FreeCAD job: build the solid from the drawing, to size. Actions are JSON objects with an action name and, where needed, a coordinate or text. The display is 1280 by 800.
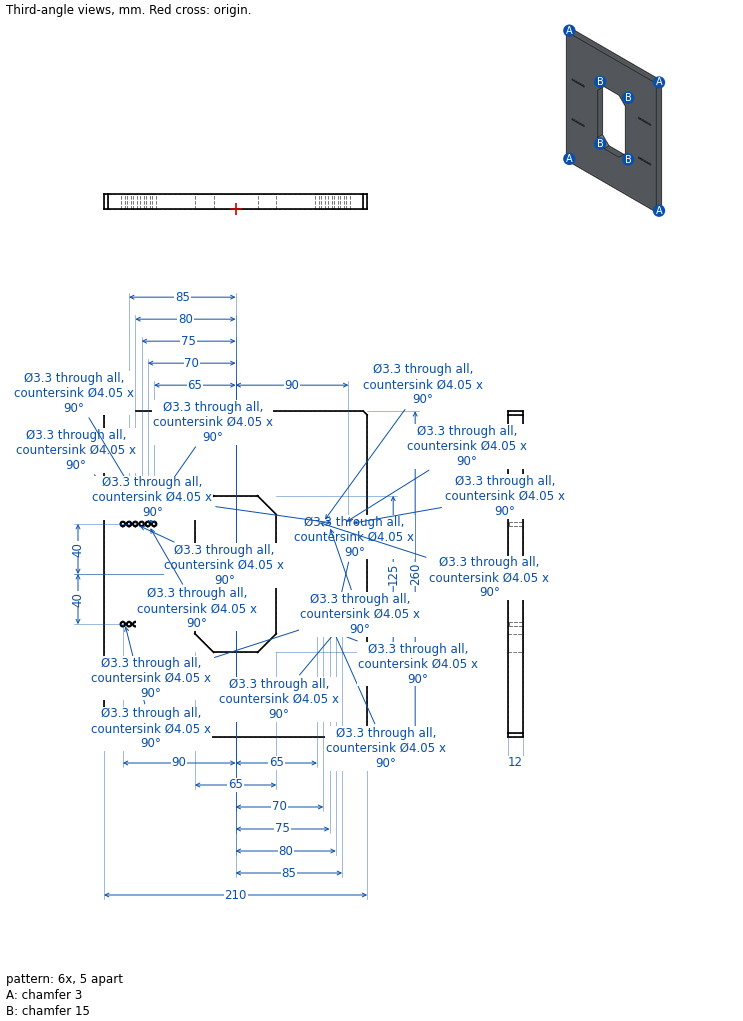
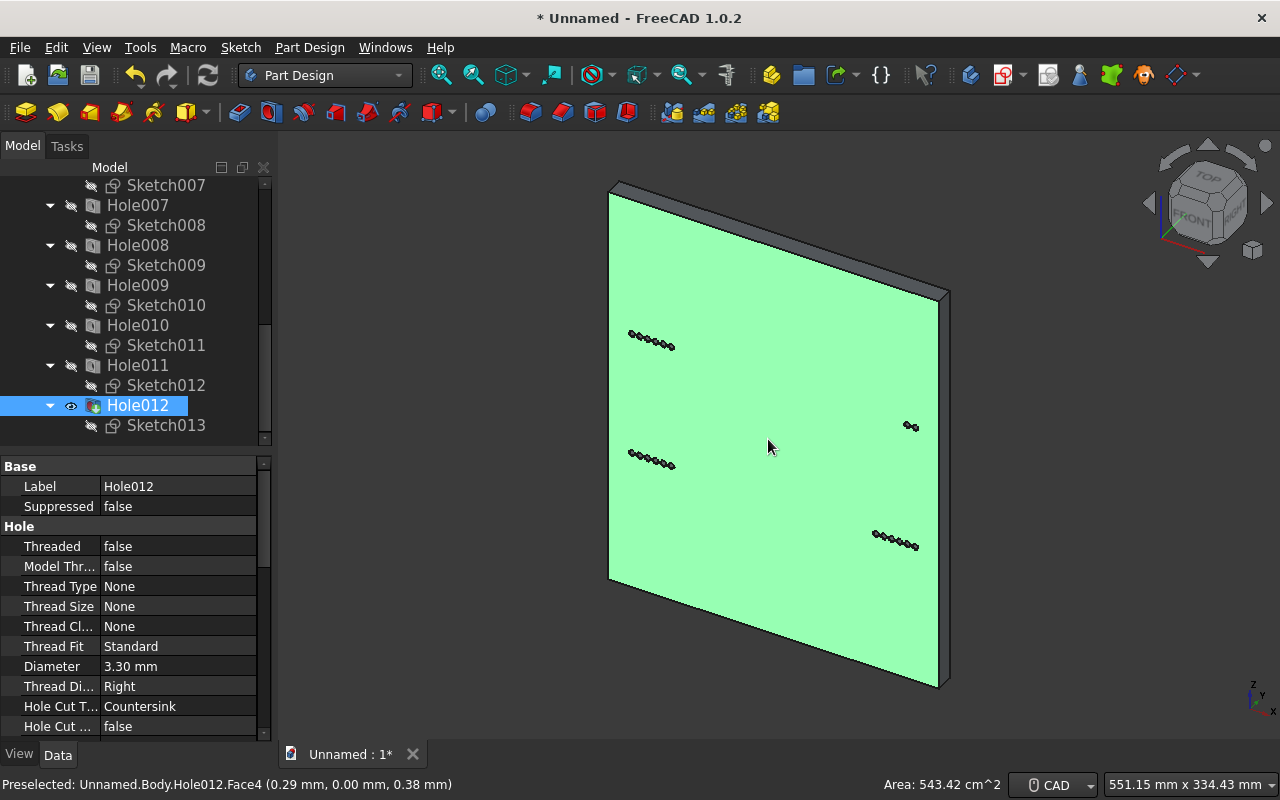
{"action": "left_click", "coordinate": [1004, 76]}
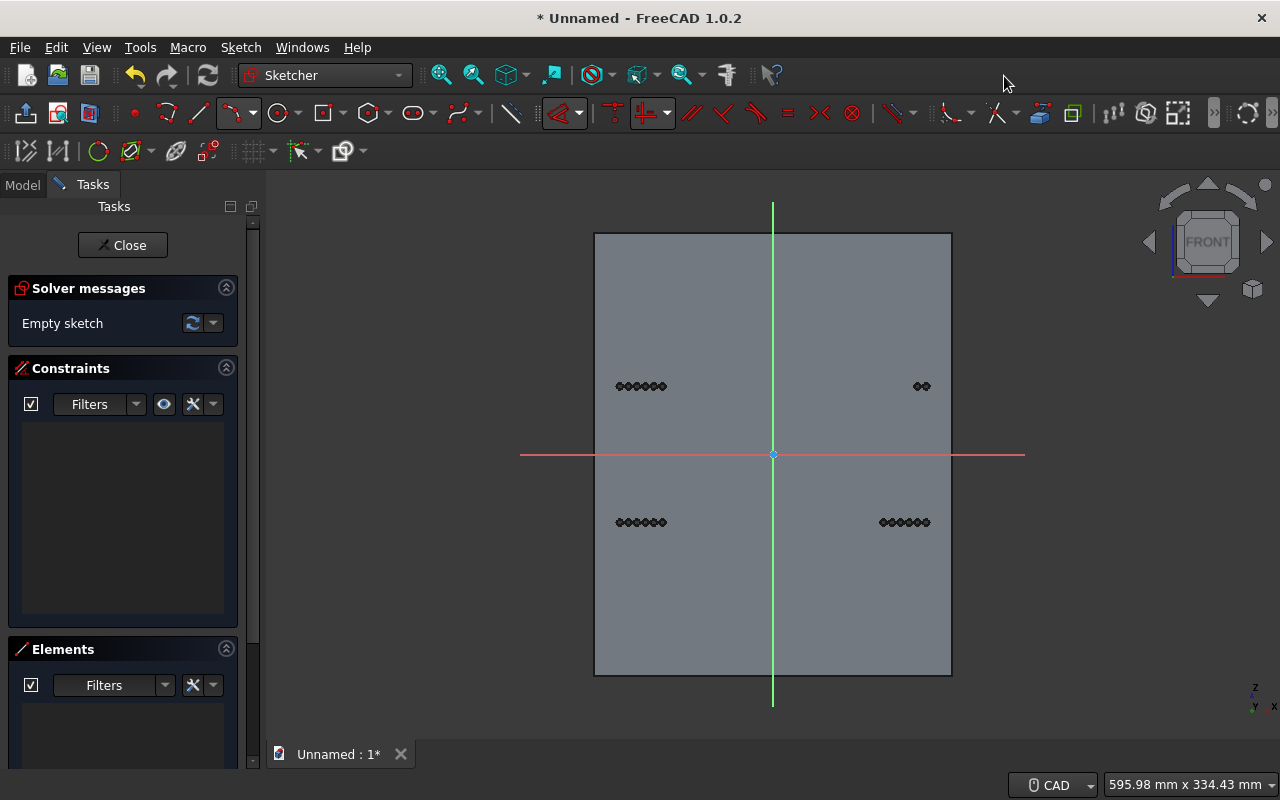
{"action": "scroll", "coordinate": [920, 383], "scroll_direction": "up", "scroll_amount": 15}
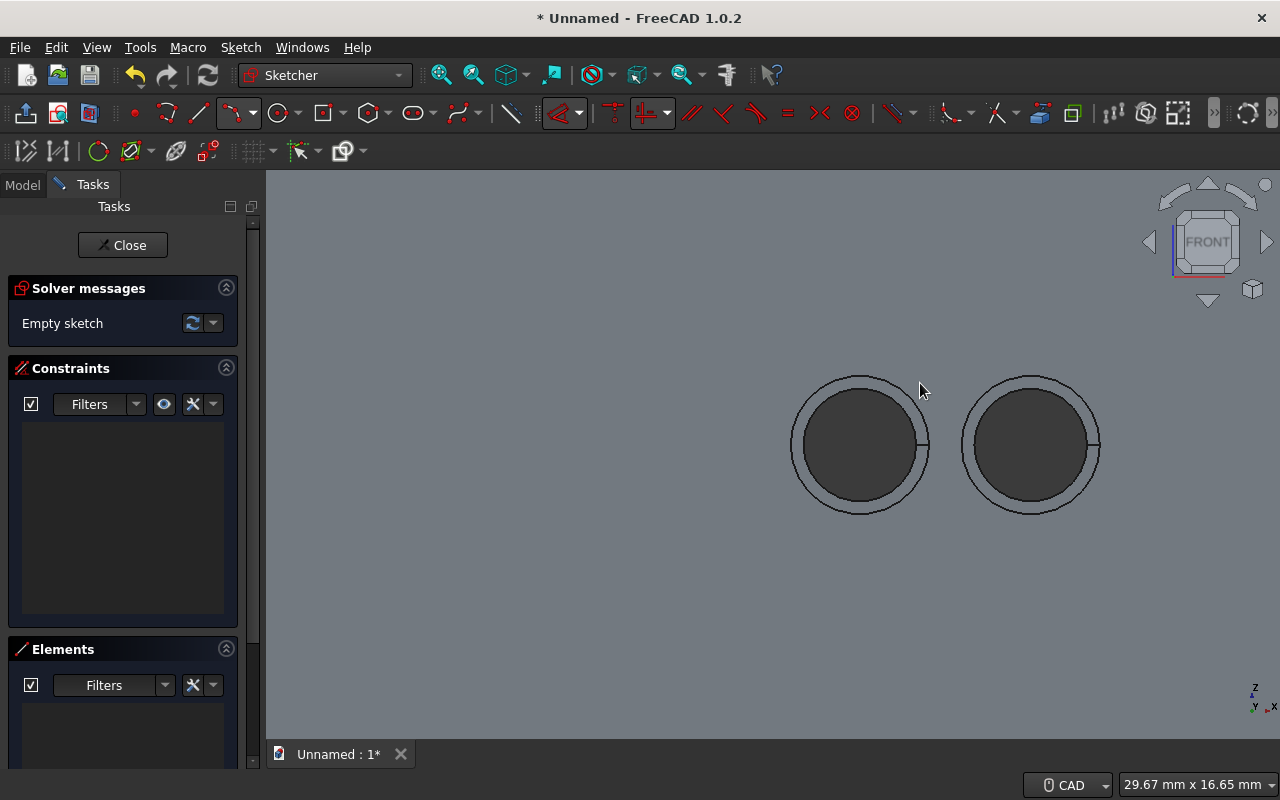
{"action": "scroll", "coordinate": [682, 441], "scroll_direction": "up", "scroll_amount": 6}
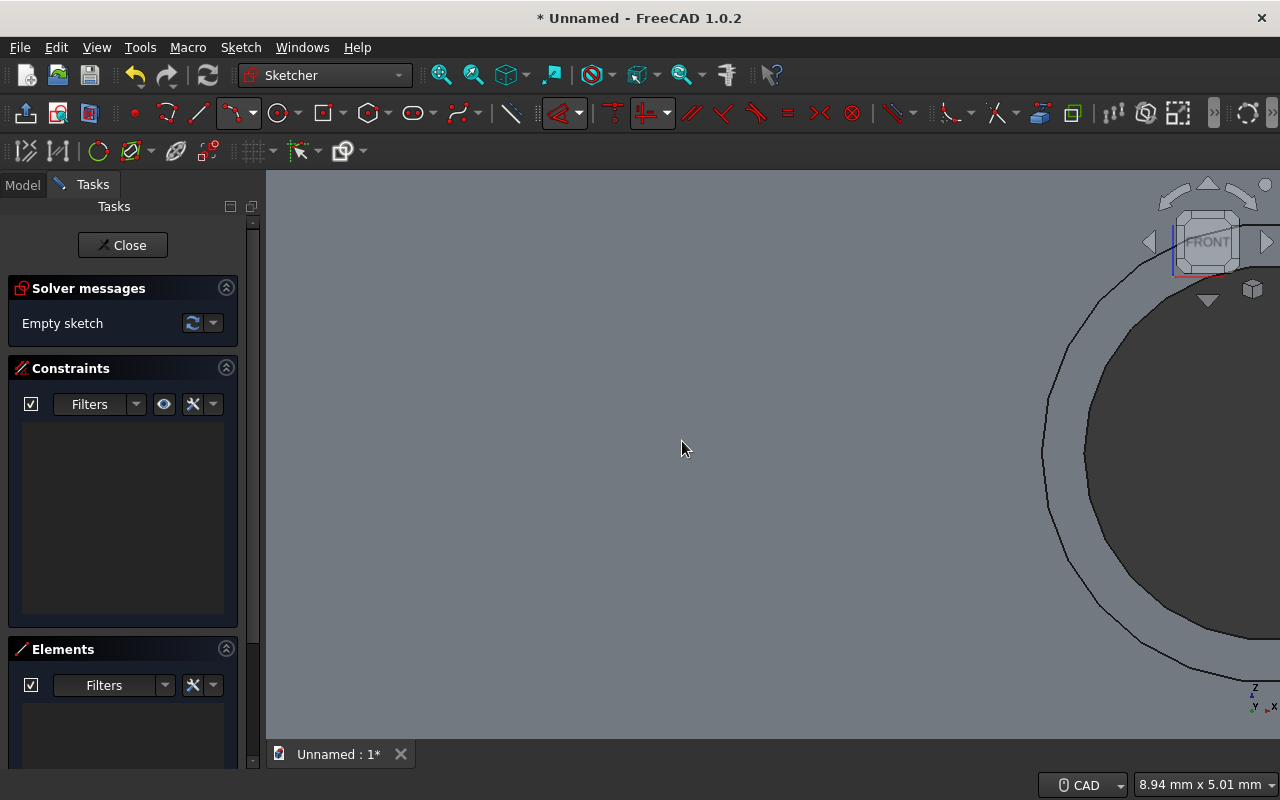
{"action": "left_click", "coordinate": [278, 114]}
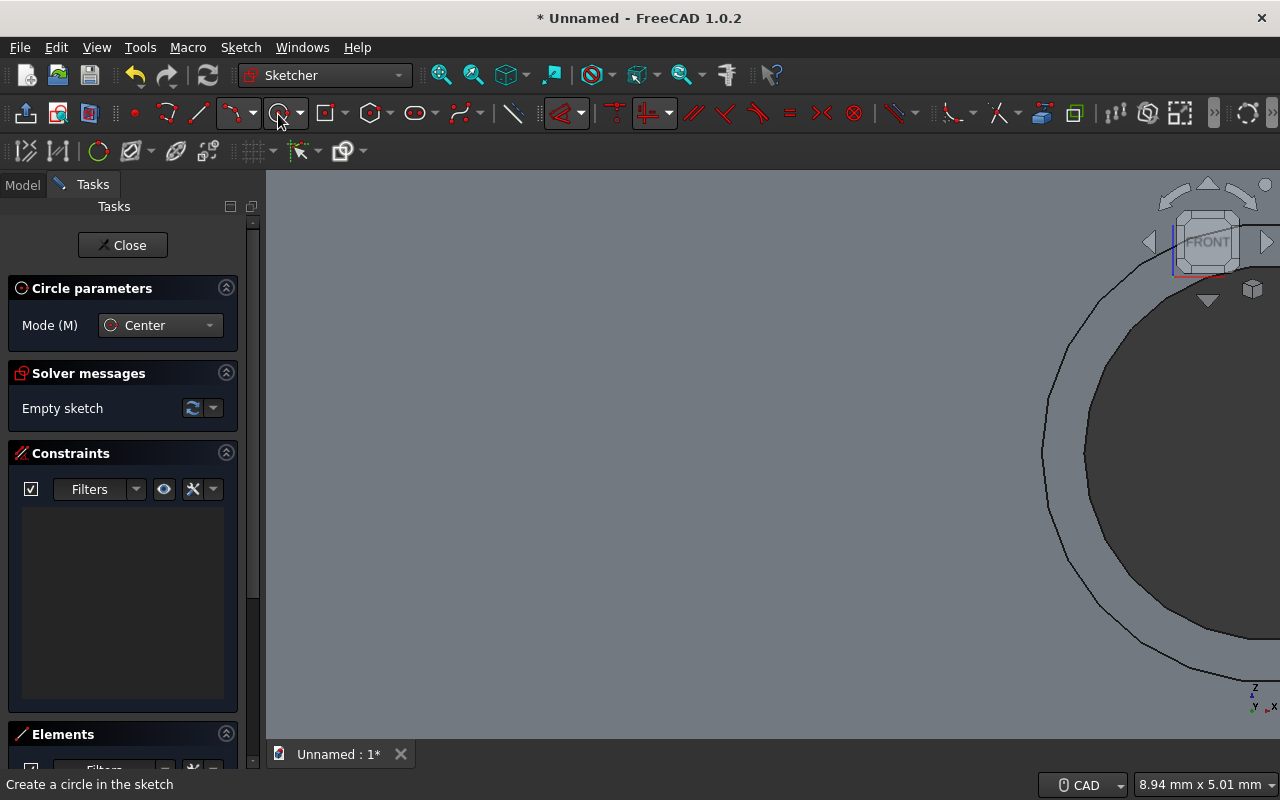
{"action": "left_click", "coordinate": [704, 453]}
{"action": "mouse_move", "coordinate": [837, 321]}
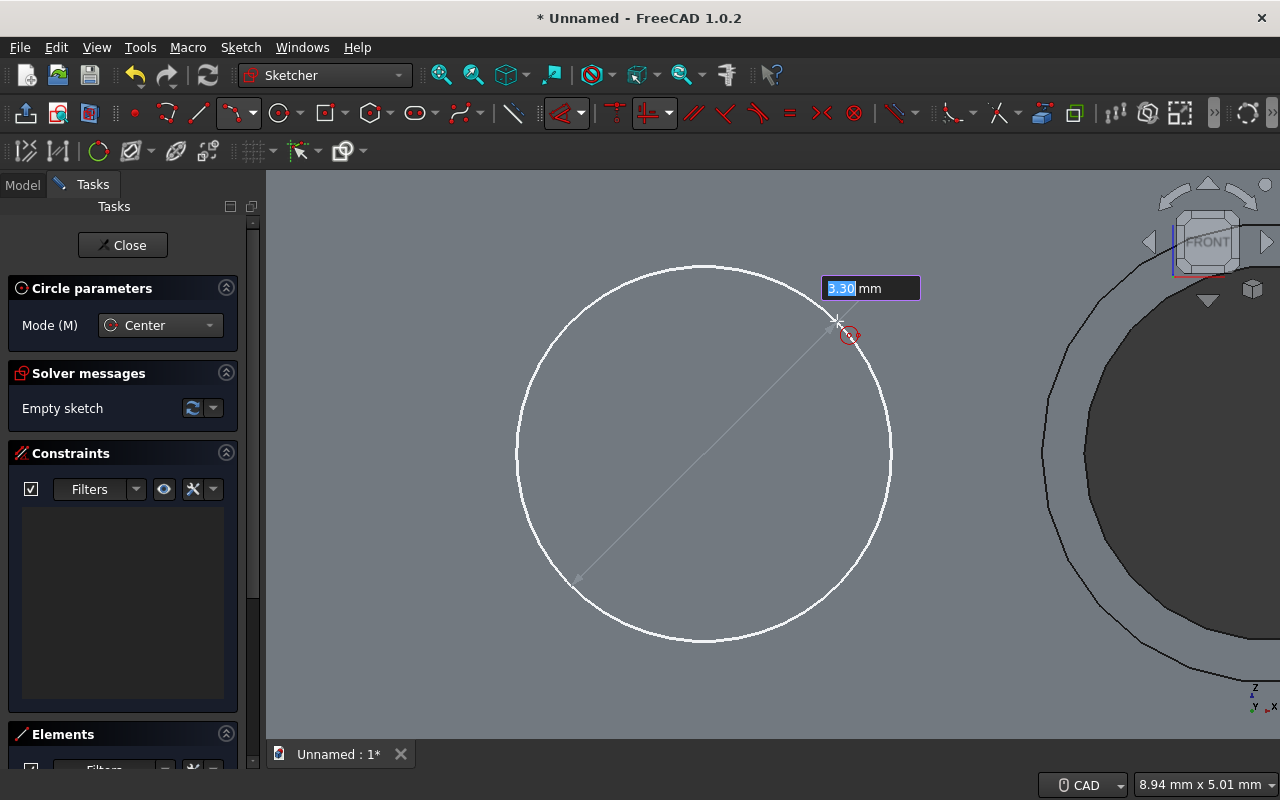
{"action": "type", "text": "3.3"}
{"action": "key", "text": "Return"}
{"action": "key", "text": "Escape"}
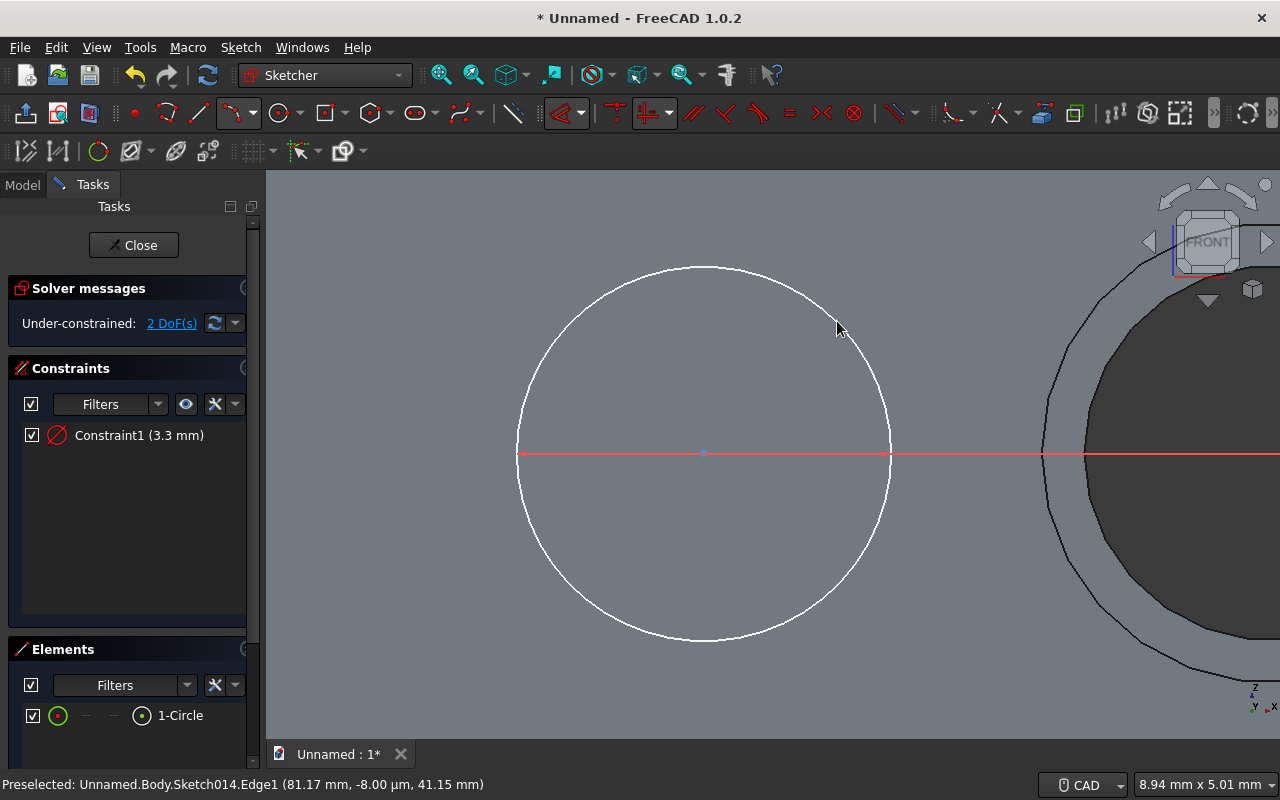
{"action": "left_click", "coordinate": [704, 454]}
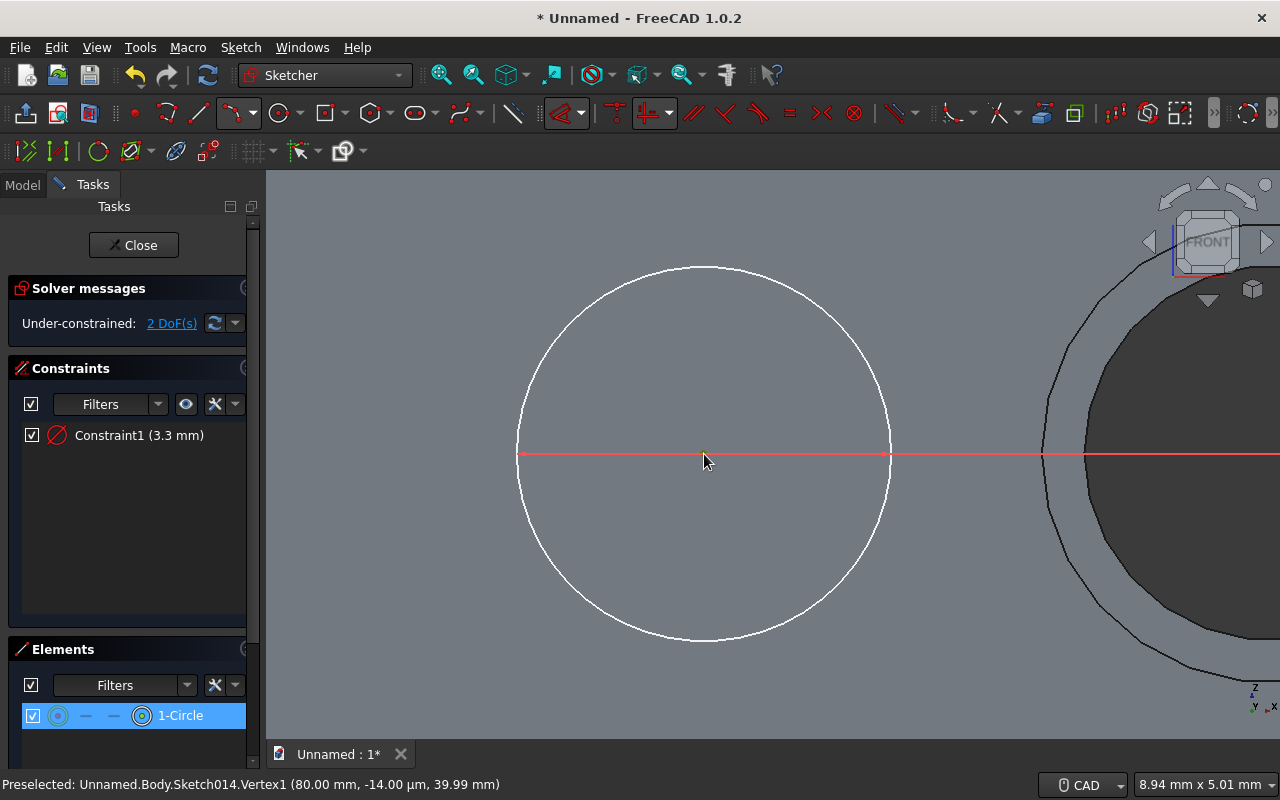
{"action": "key", "text": "l"}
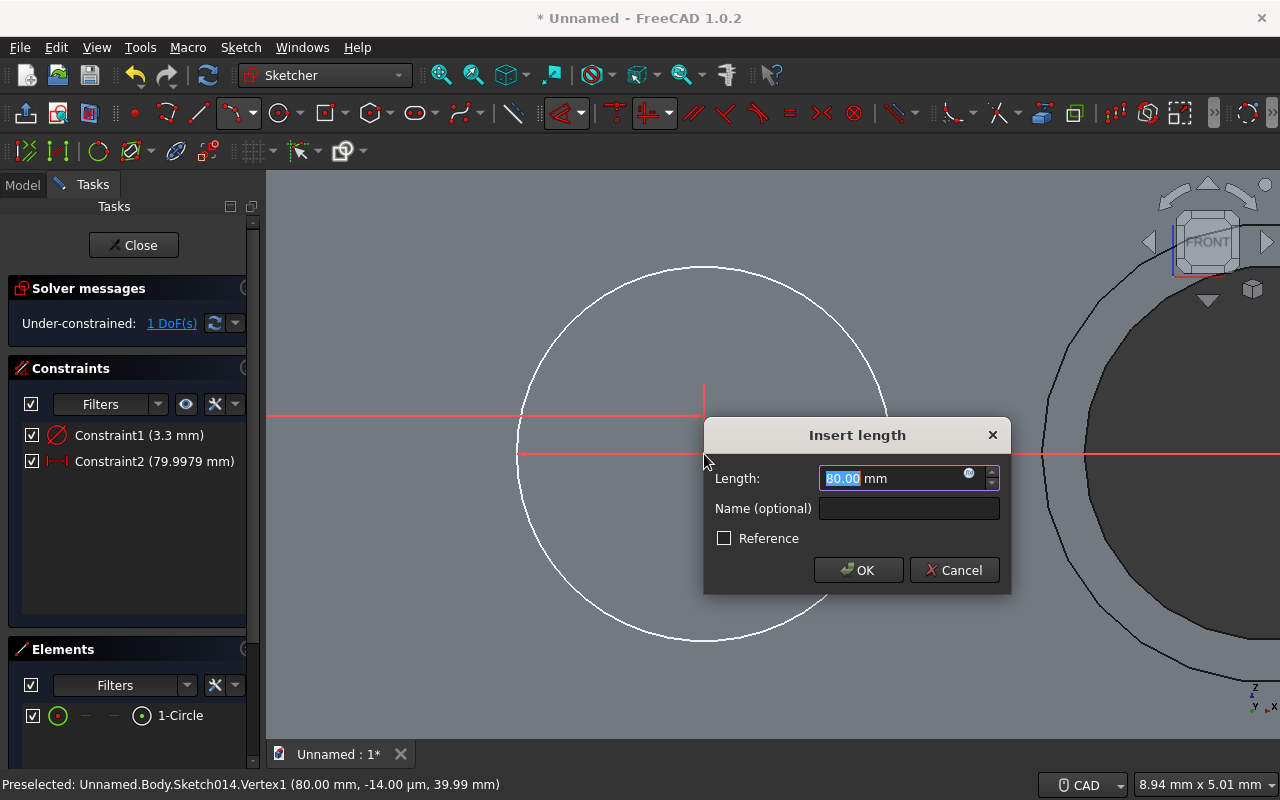
{"action": "type", "text": "80"}
{"action": "key", "text": "Return"}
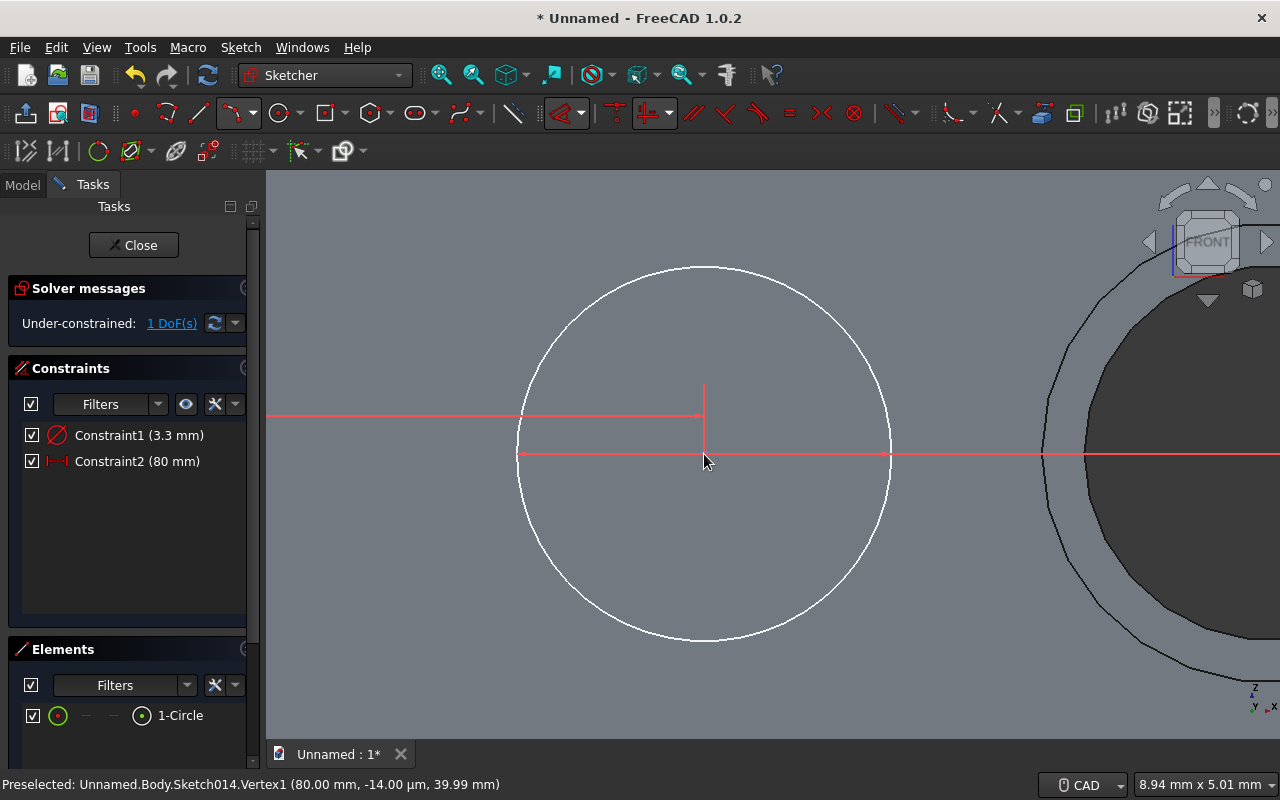
{"action": "left_click", "coordinate": [704, 454]}